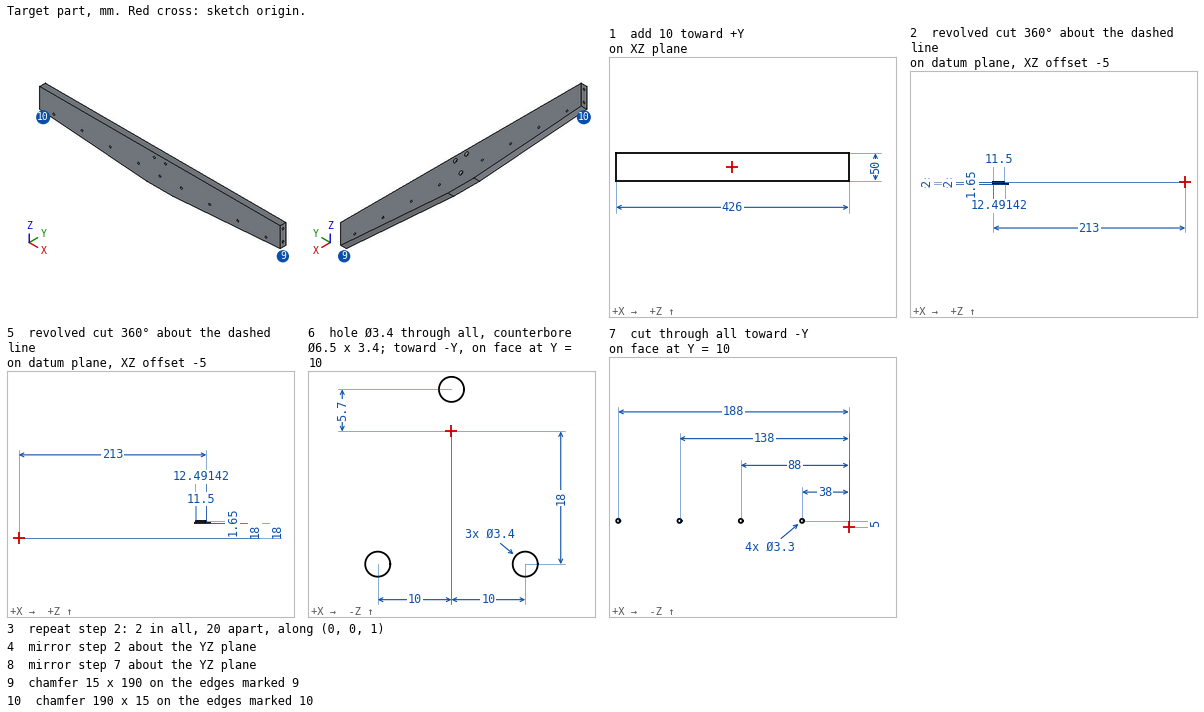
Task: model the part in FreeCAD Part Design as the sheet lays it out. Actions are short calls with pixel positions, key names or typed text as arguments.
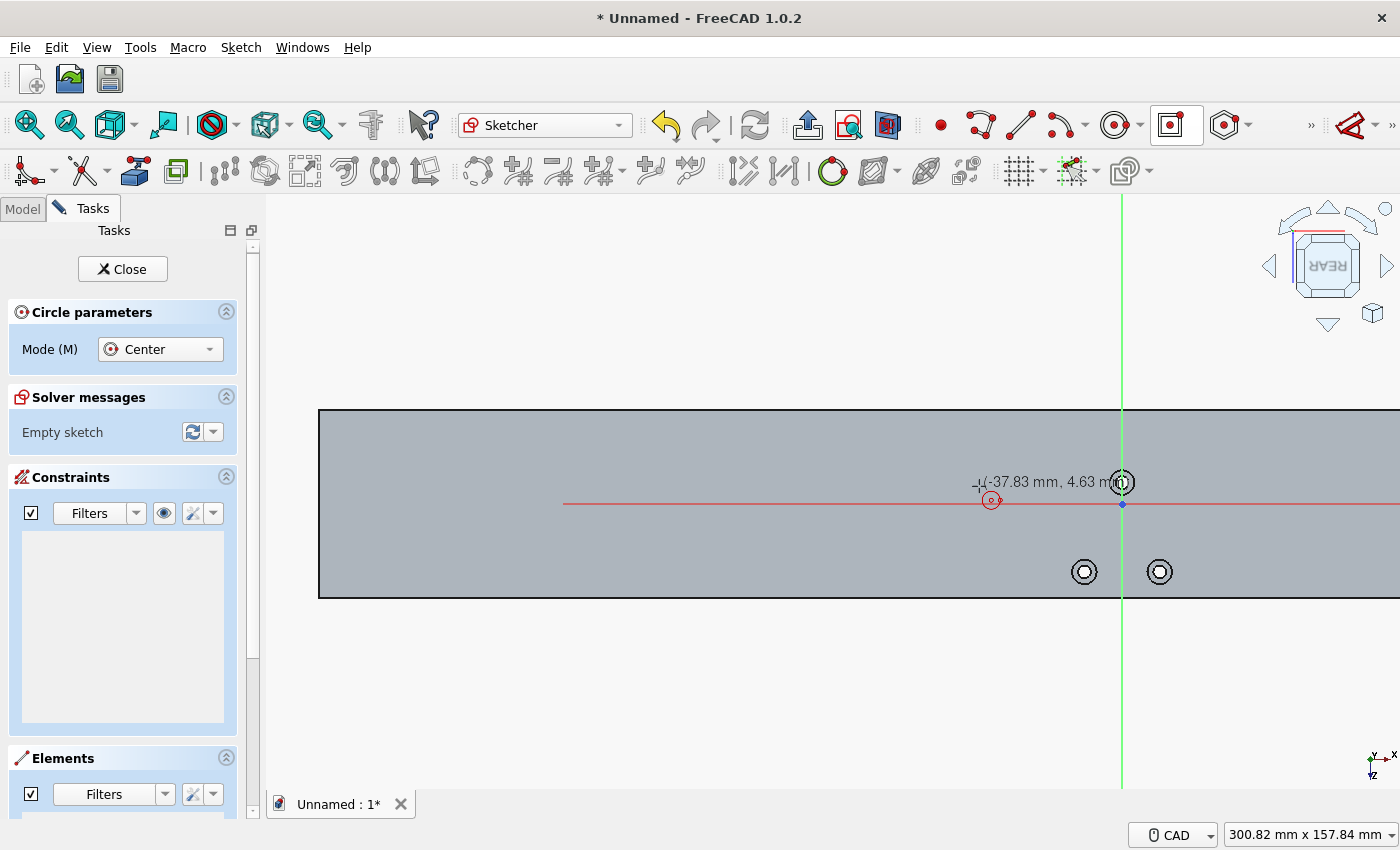
click(979, 485)
move(983, 481)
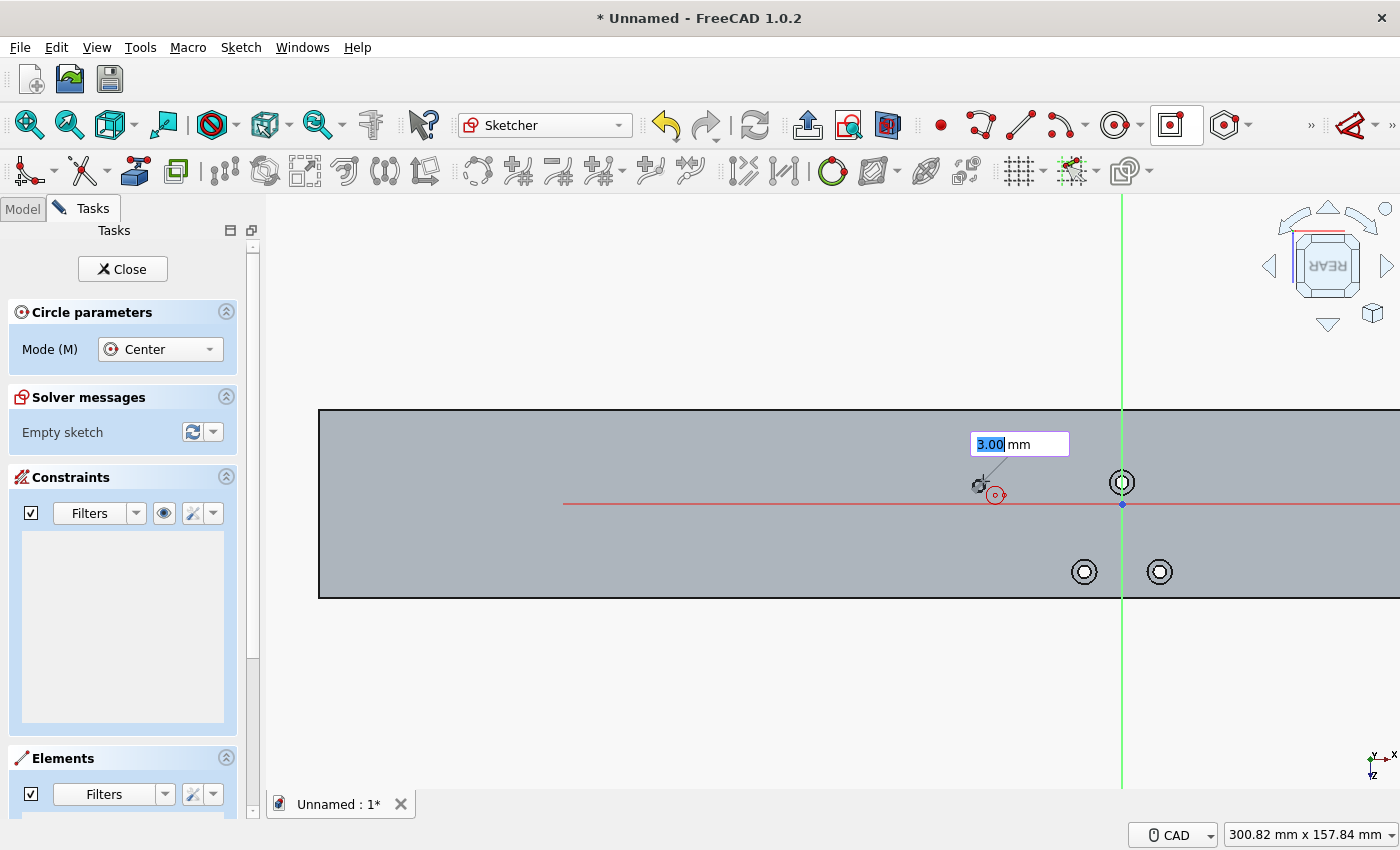
text(3.3)
key(Return)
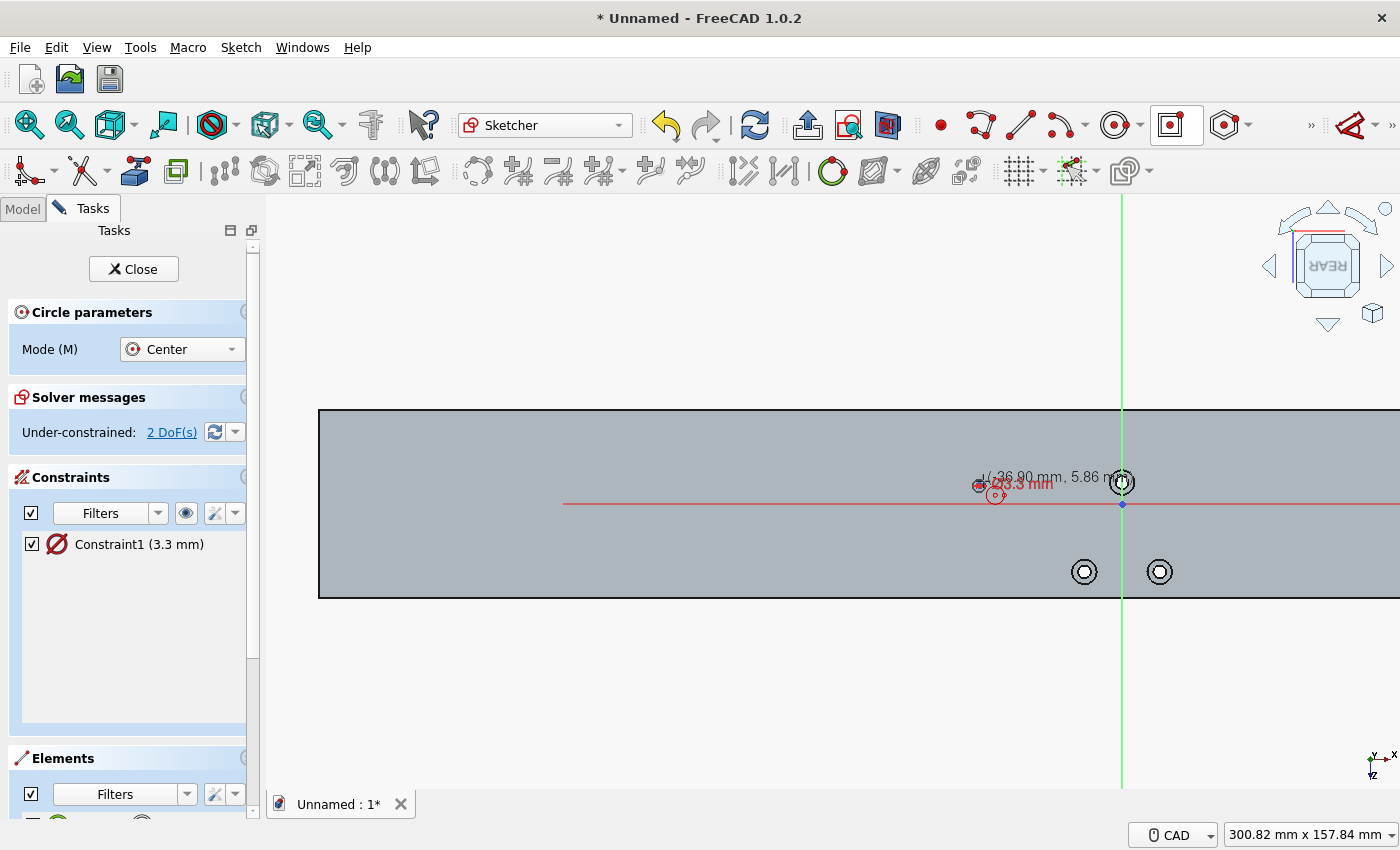
scroll(790, 485, up, 7)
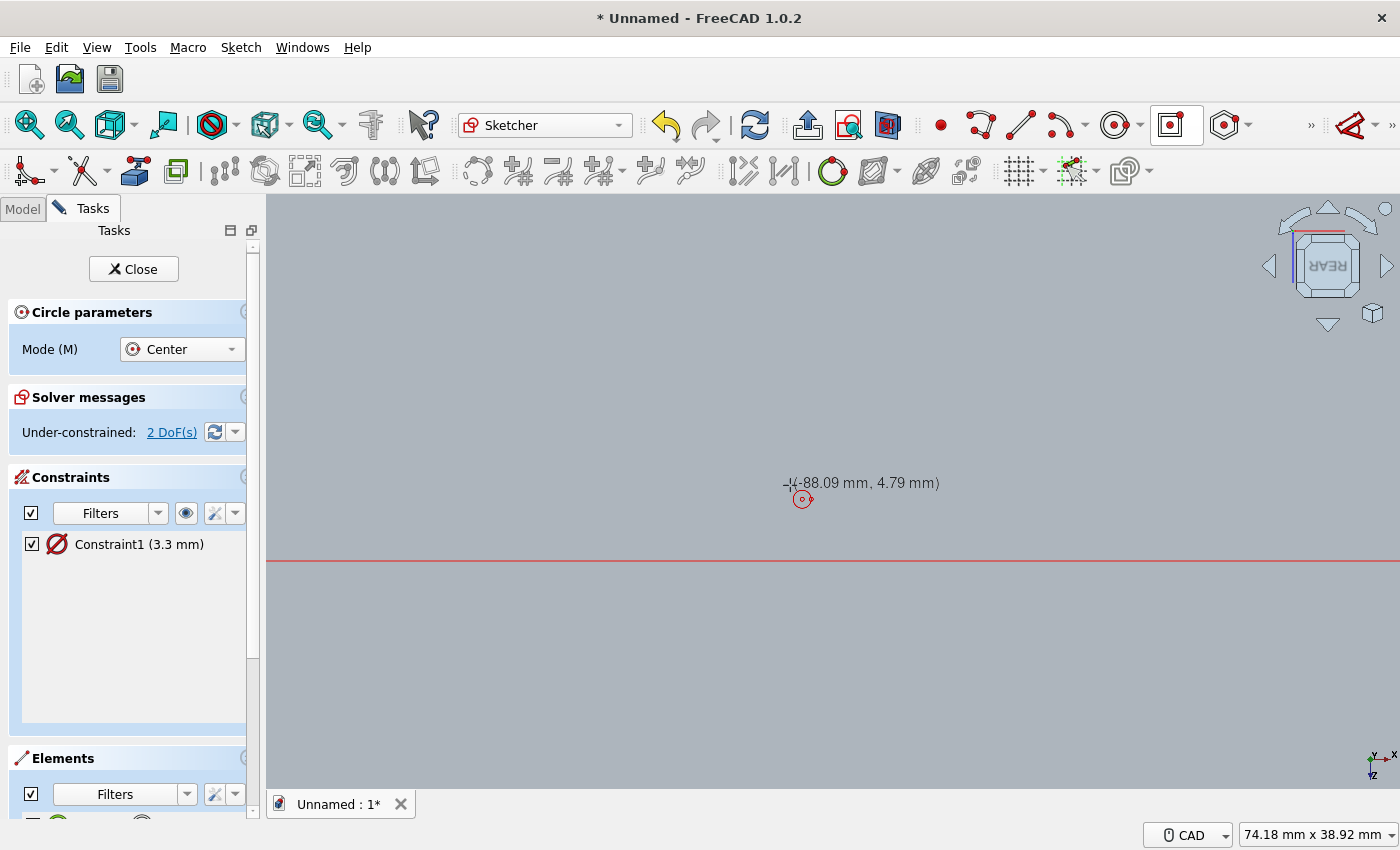
scroll(790, 485, down, 7)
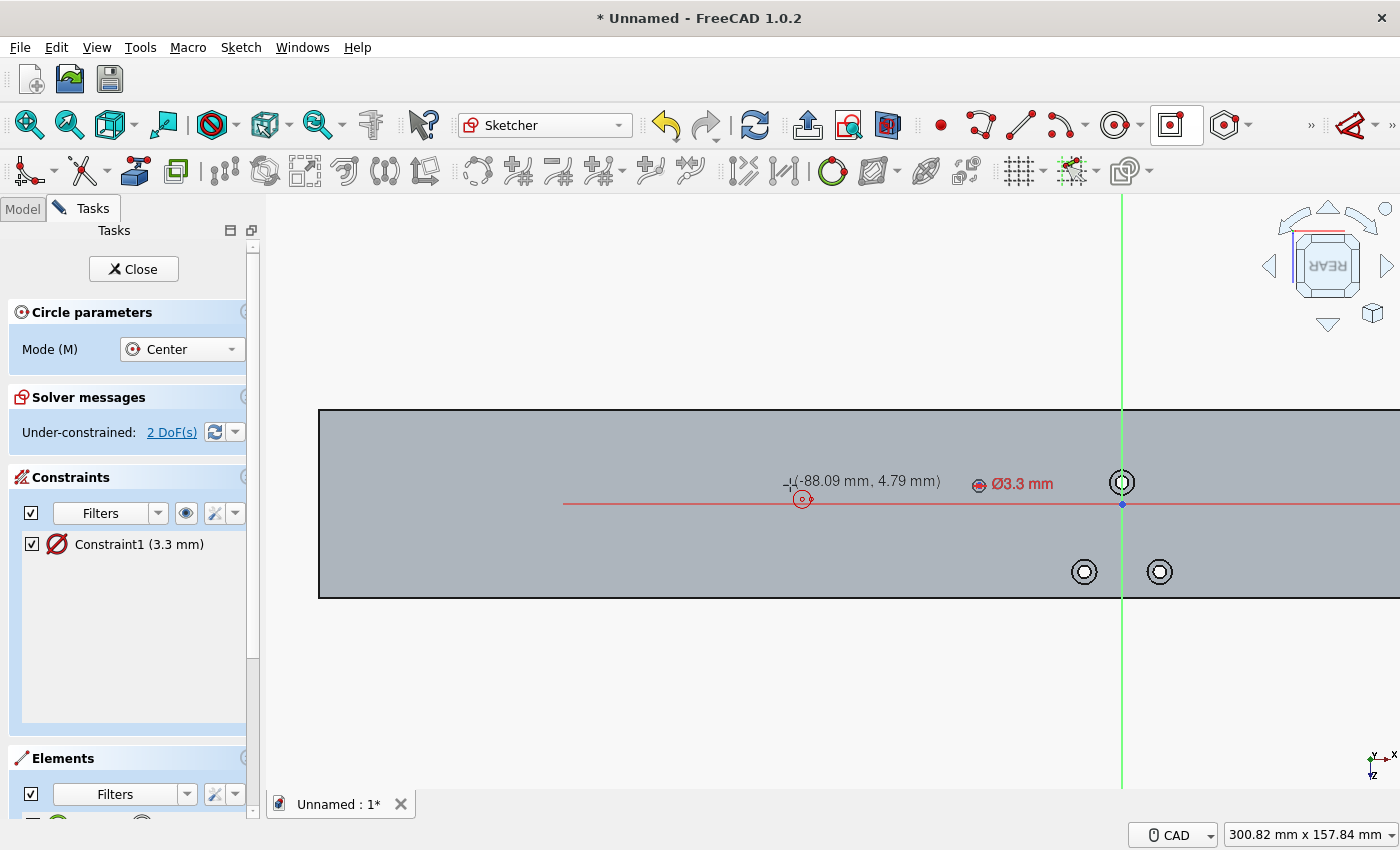
click(790, 485)
move(795, 481)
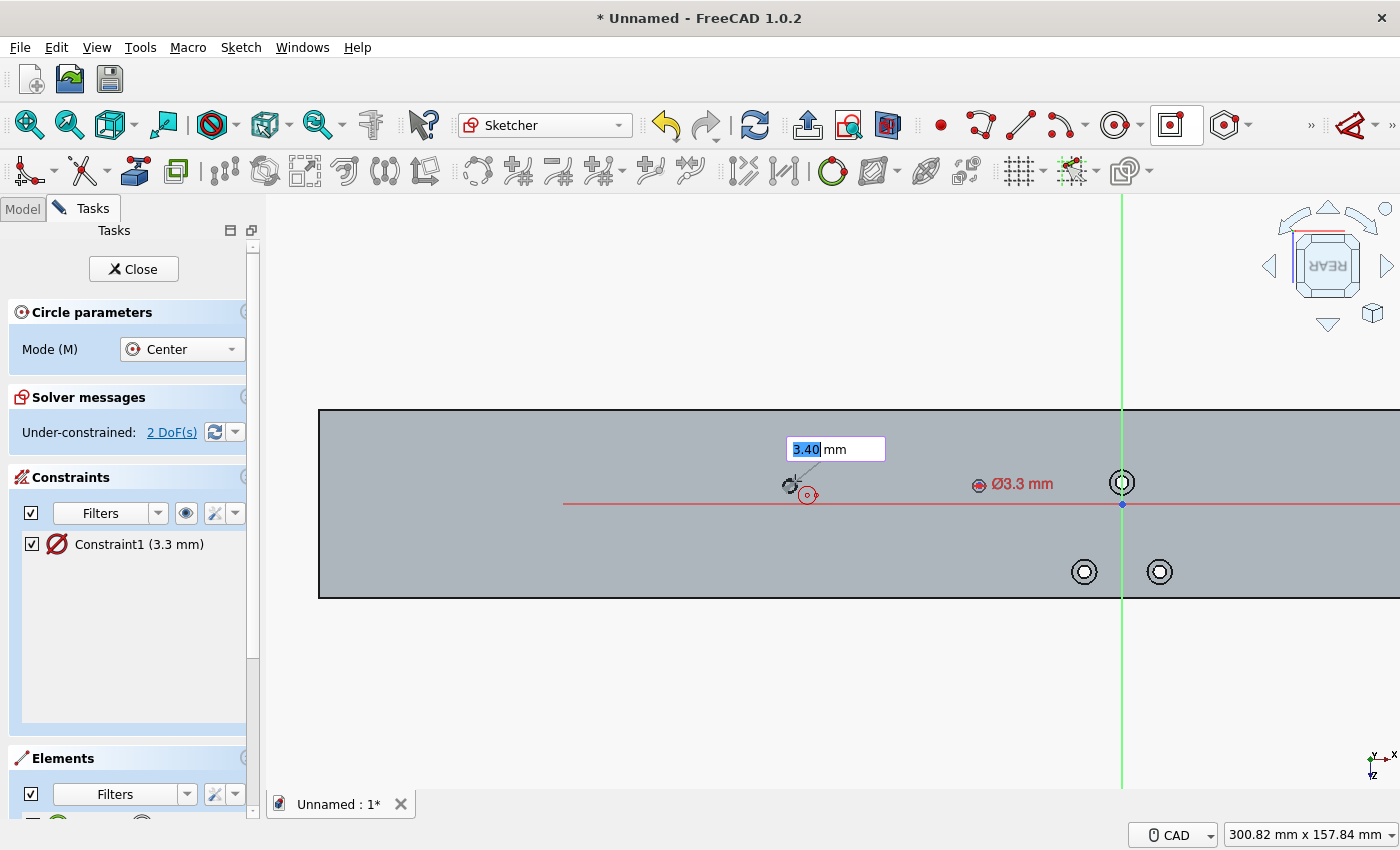
text(3.3)
key(Return)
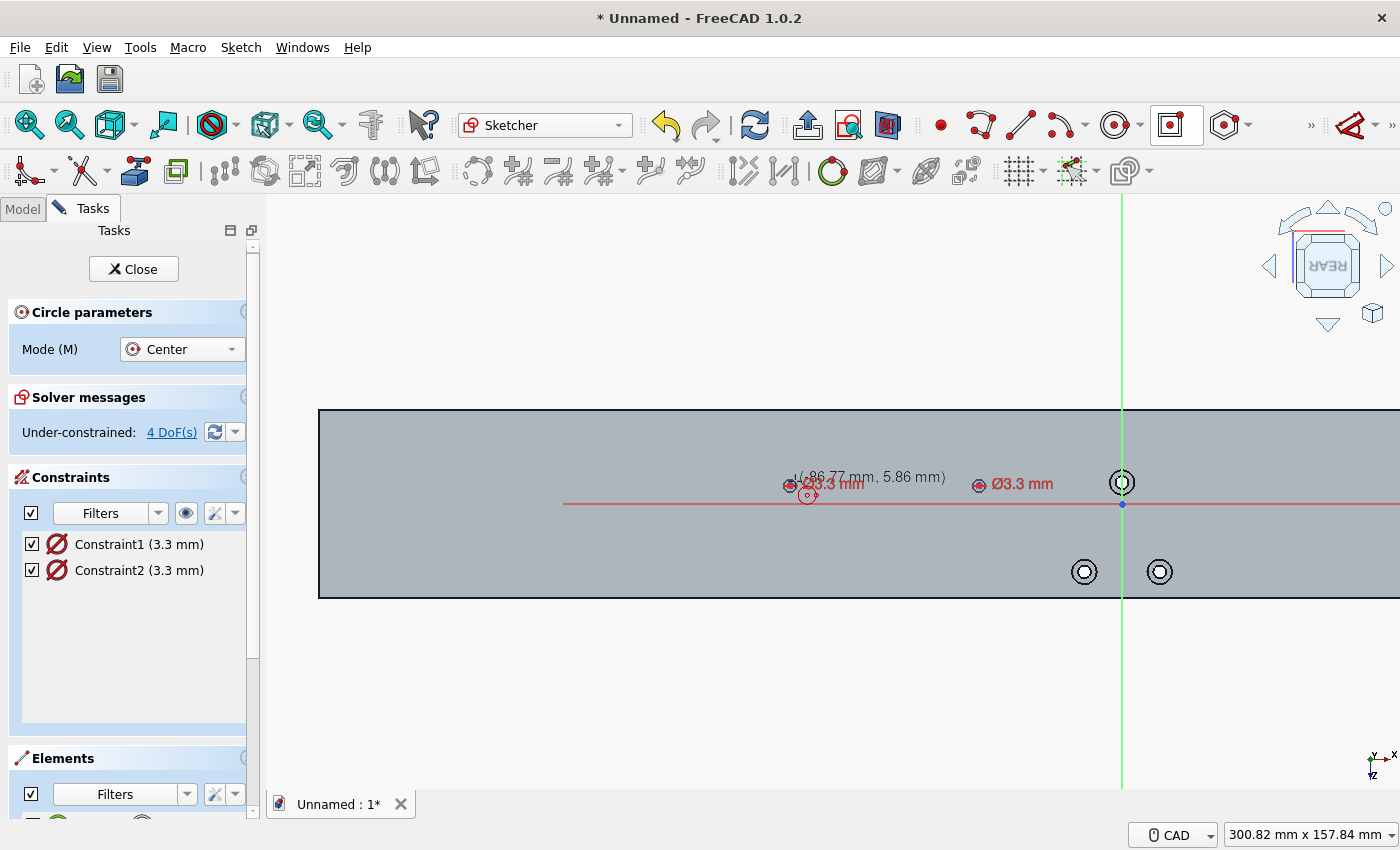
scroll(602, 485, up, 7)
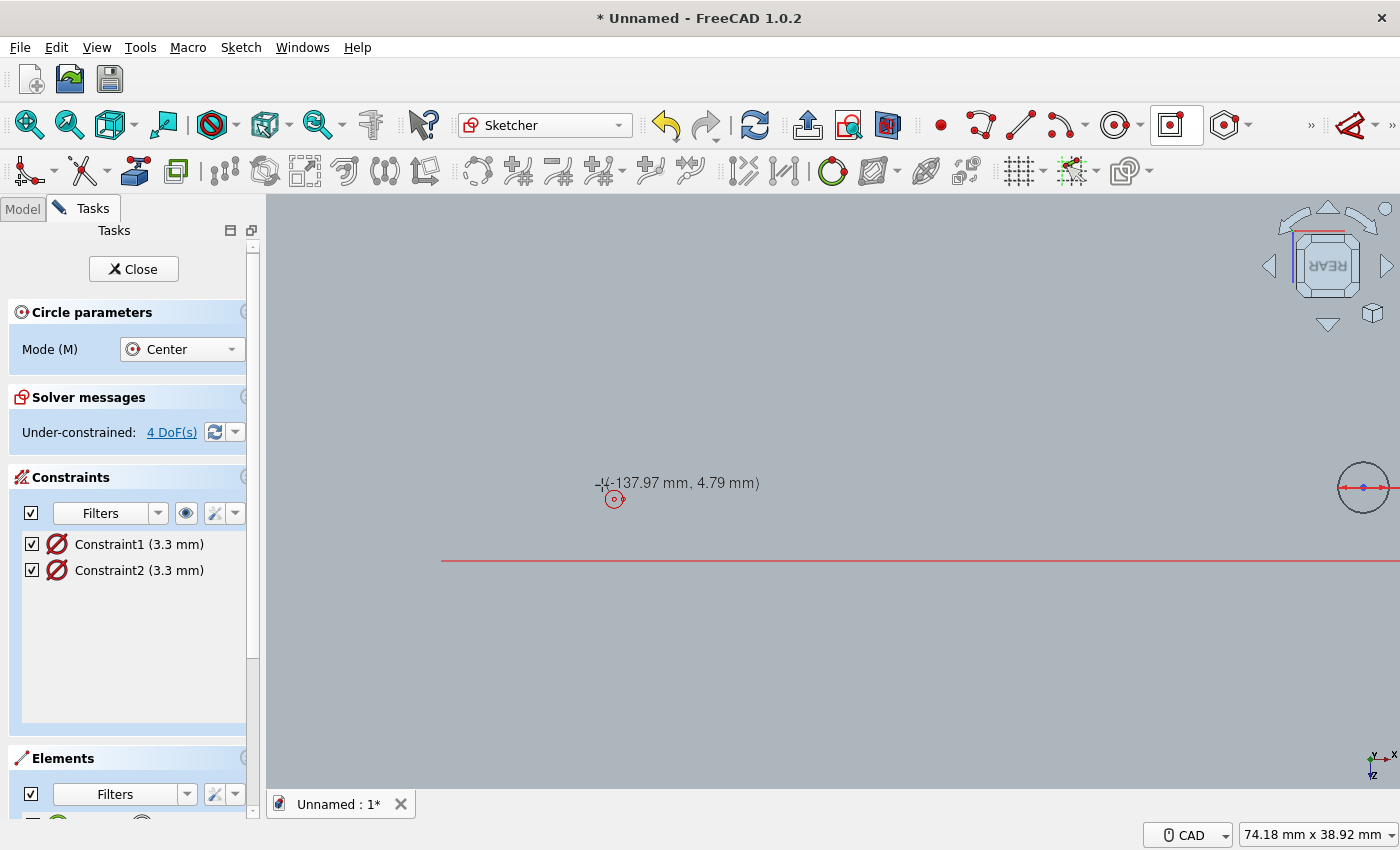
scroll(602, 485, down, 7)